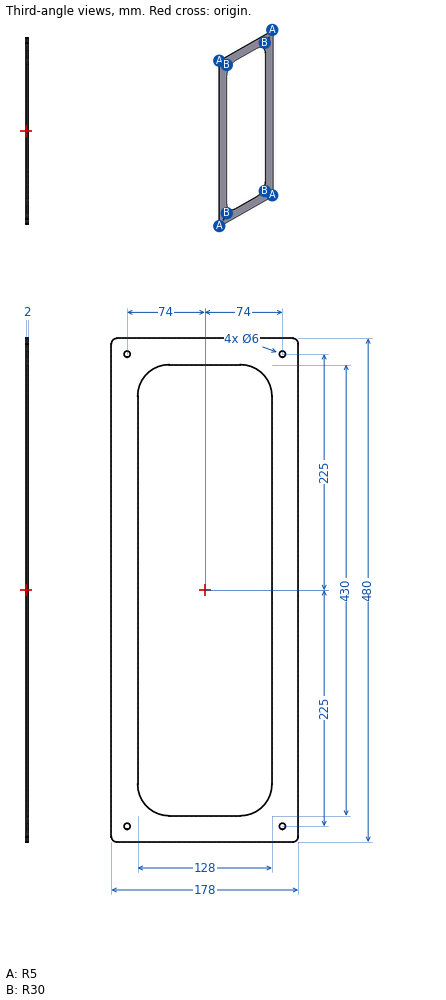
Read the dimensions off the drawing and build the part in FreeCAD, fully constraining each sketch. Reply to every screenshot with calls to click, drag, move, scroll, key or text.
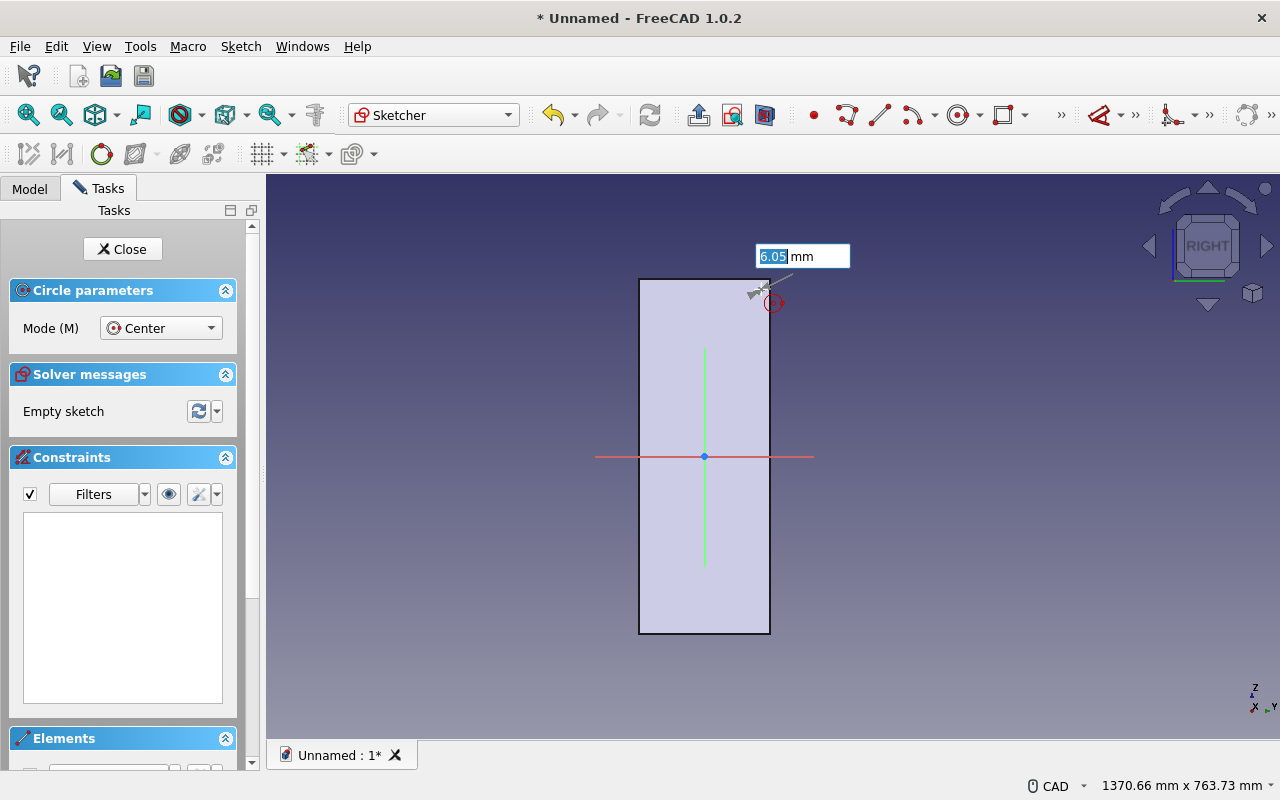
text(6)
key(Return)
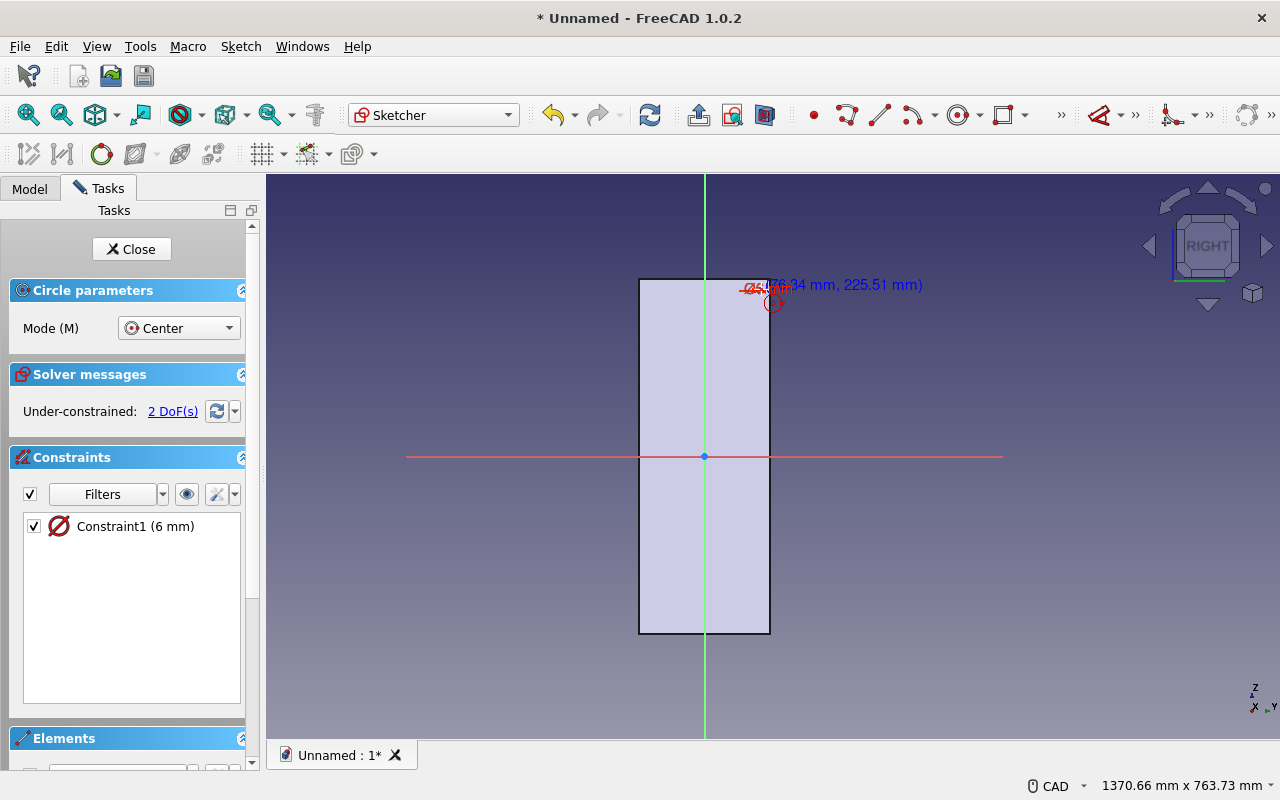
scroll(759, 623, up, 12)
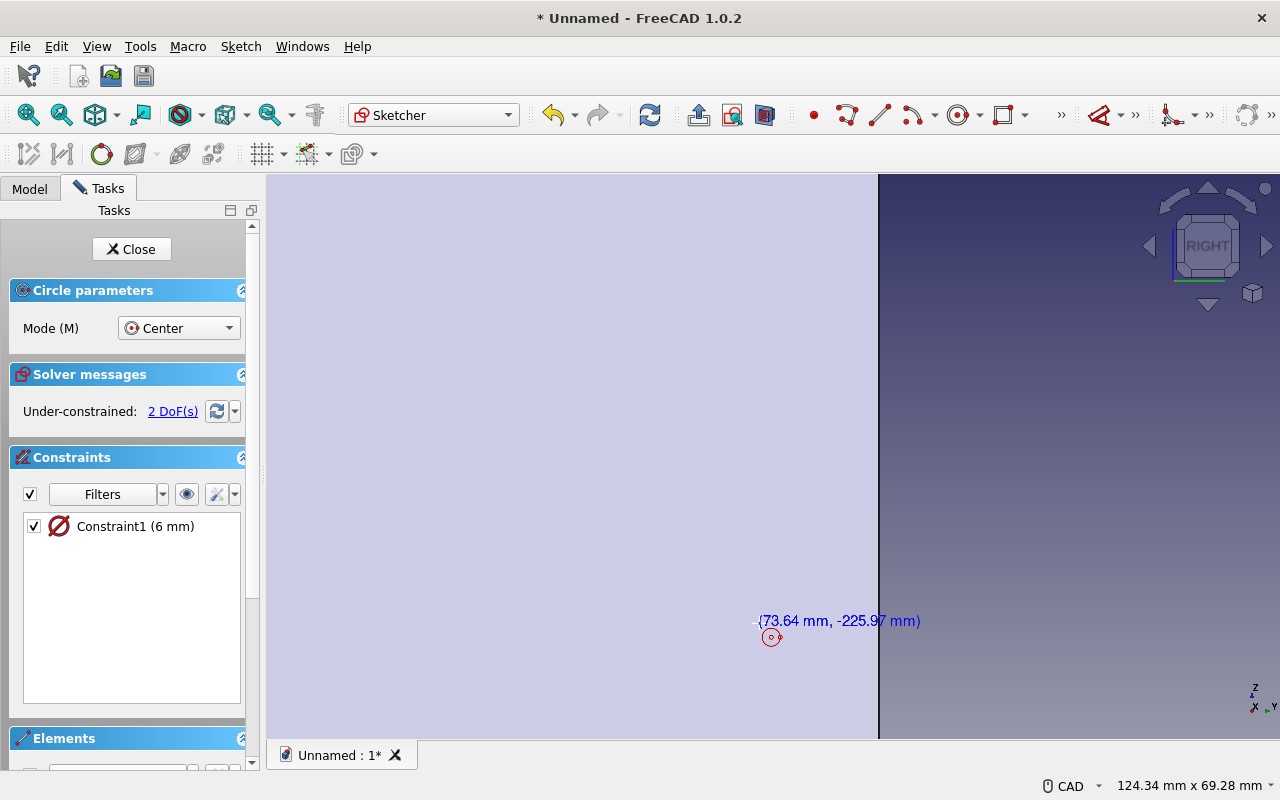
scroll(759, 623, down, 12)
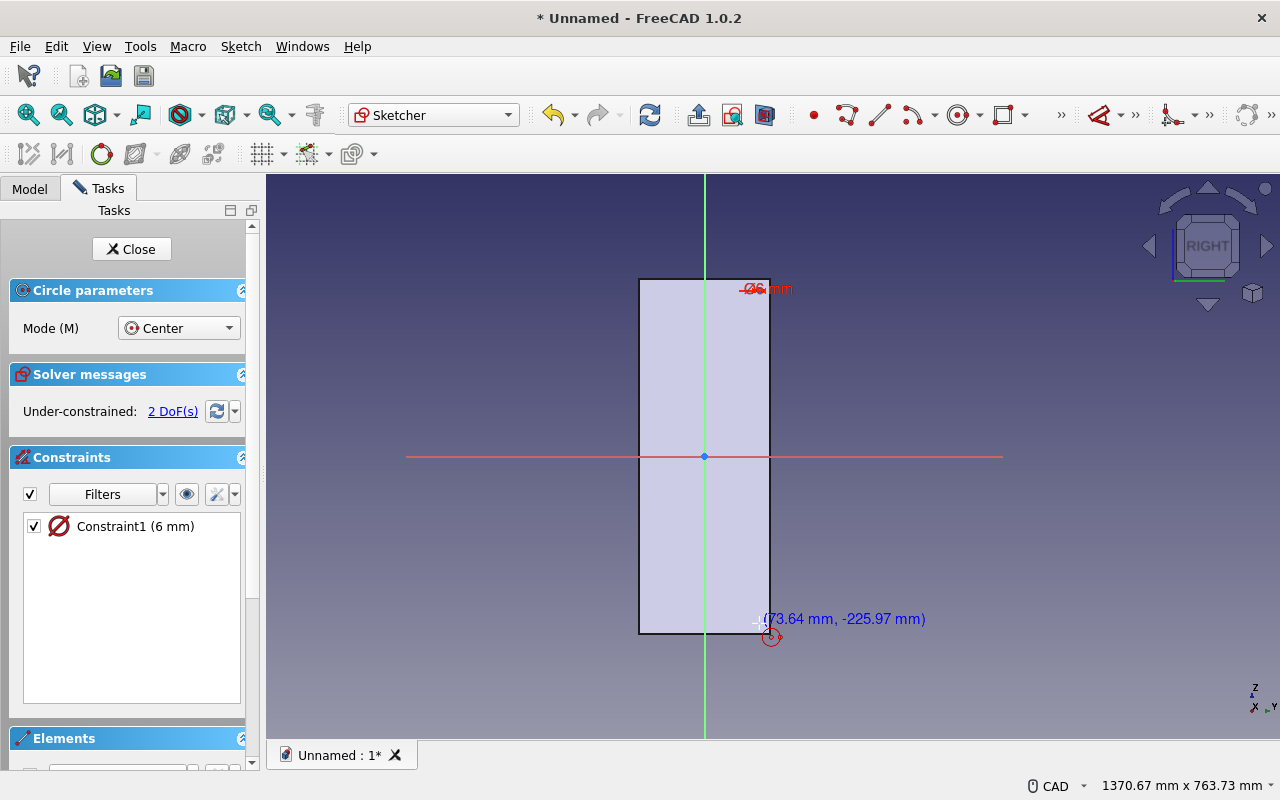
click(759, 623)
move(761, 622)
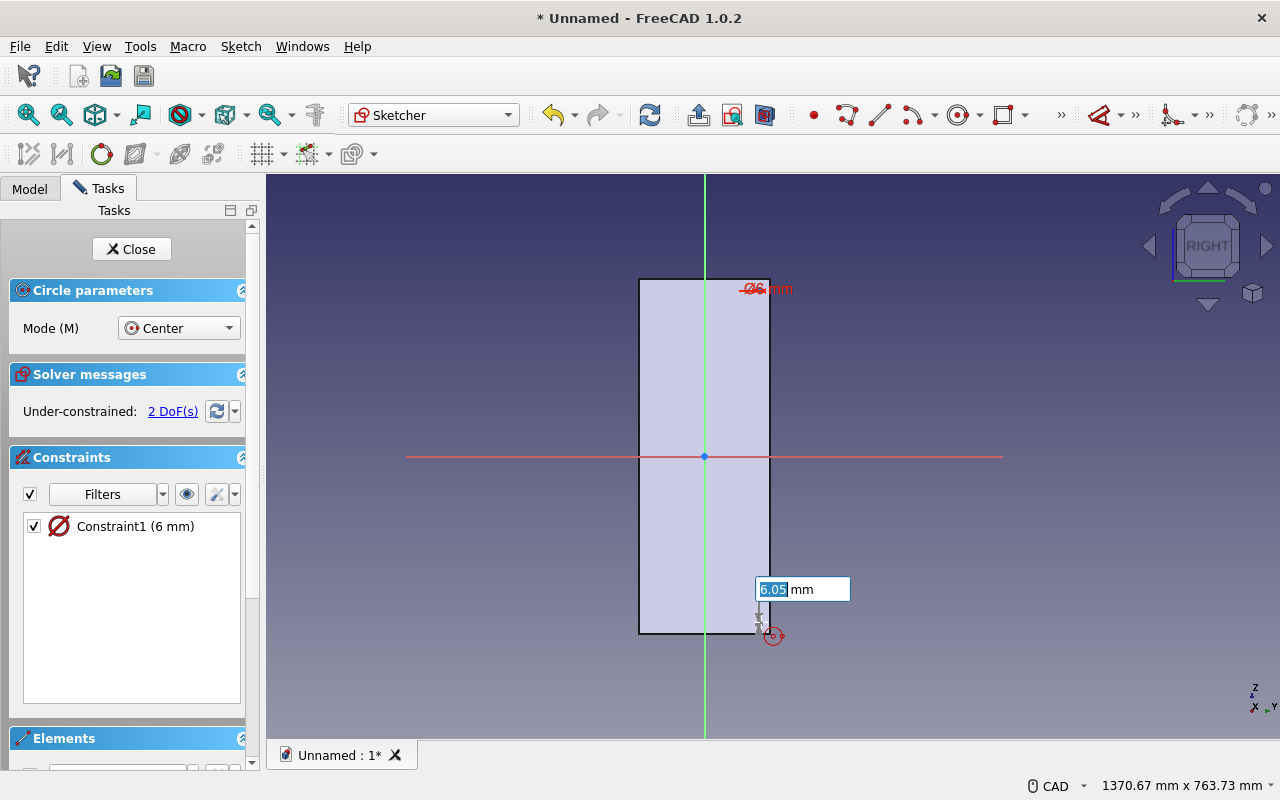
text(6)
key(Return)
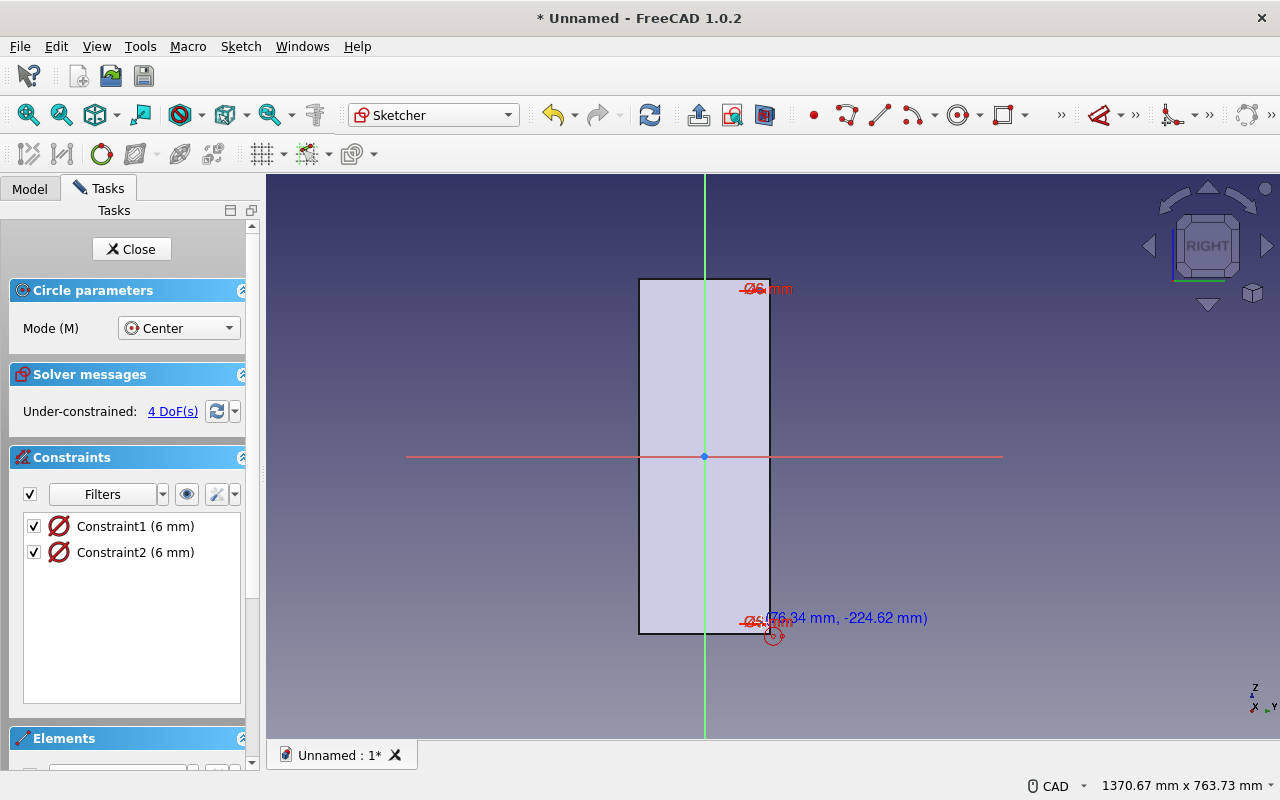
scroll(650, 290, up, 12)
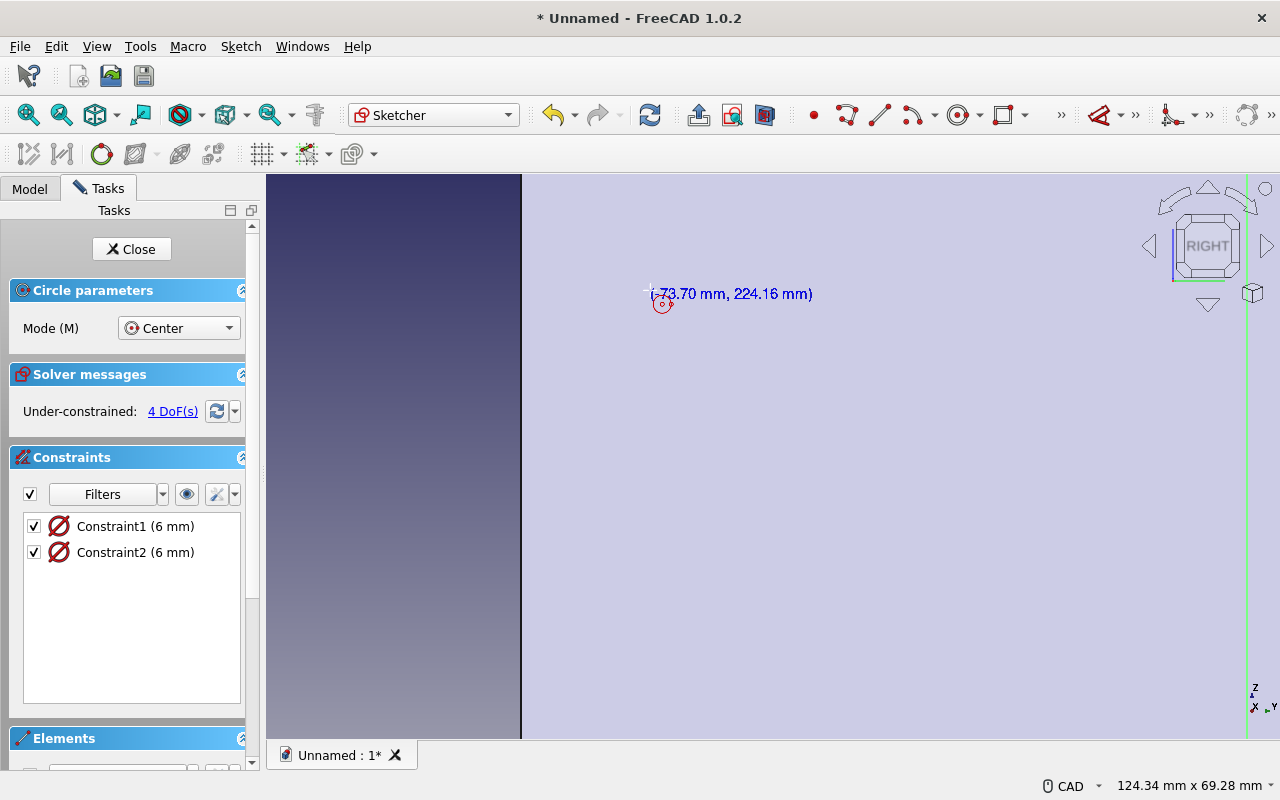
scroll(650, 290, down, 12)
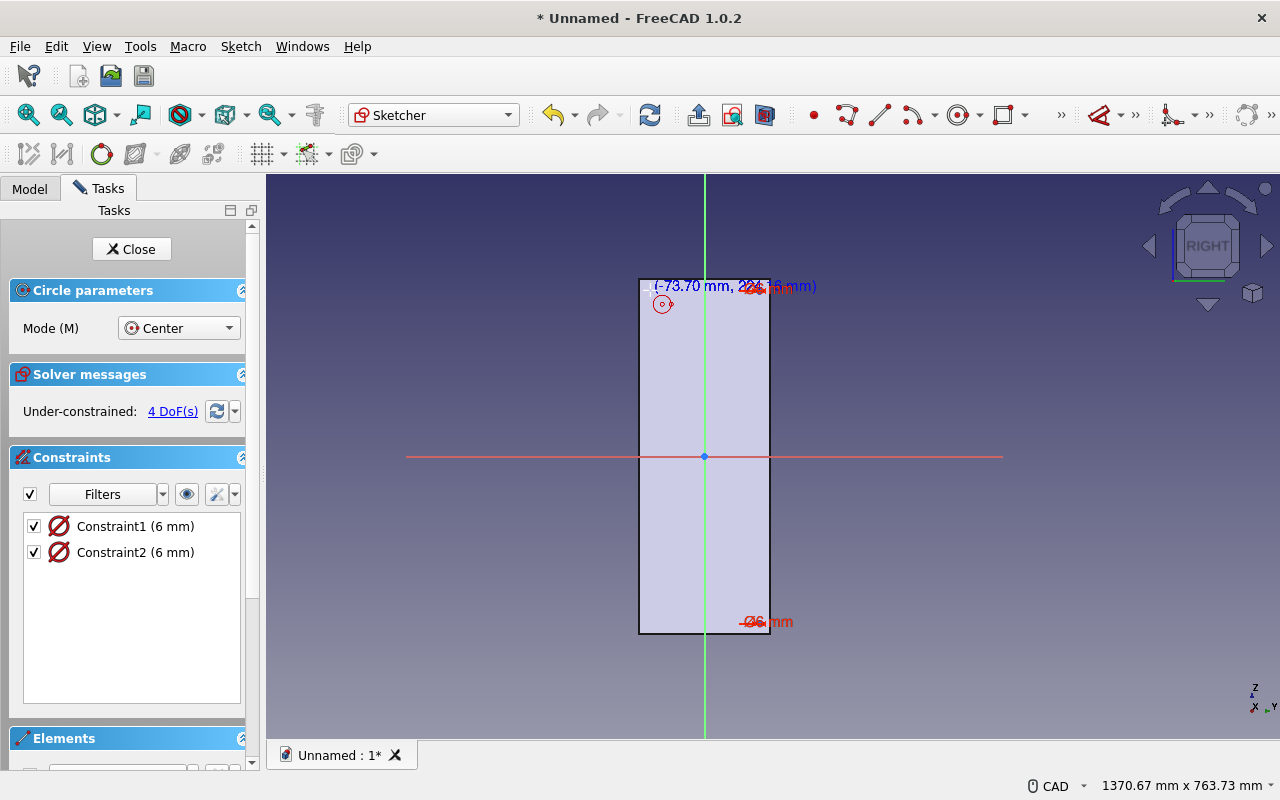
click(650, 290)
move(651, 289)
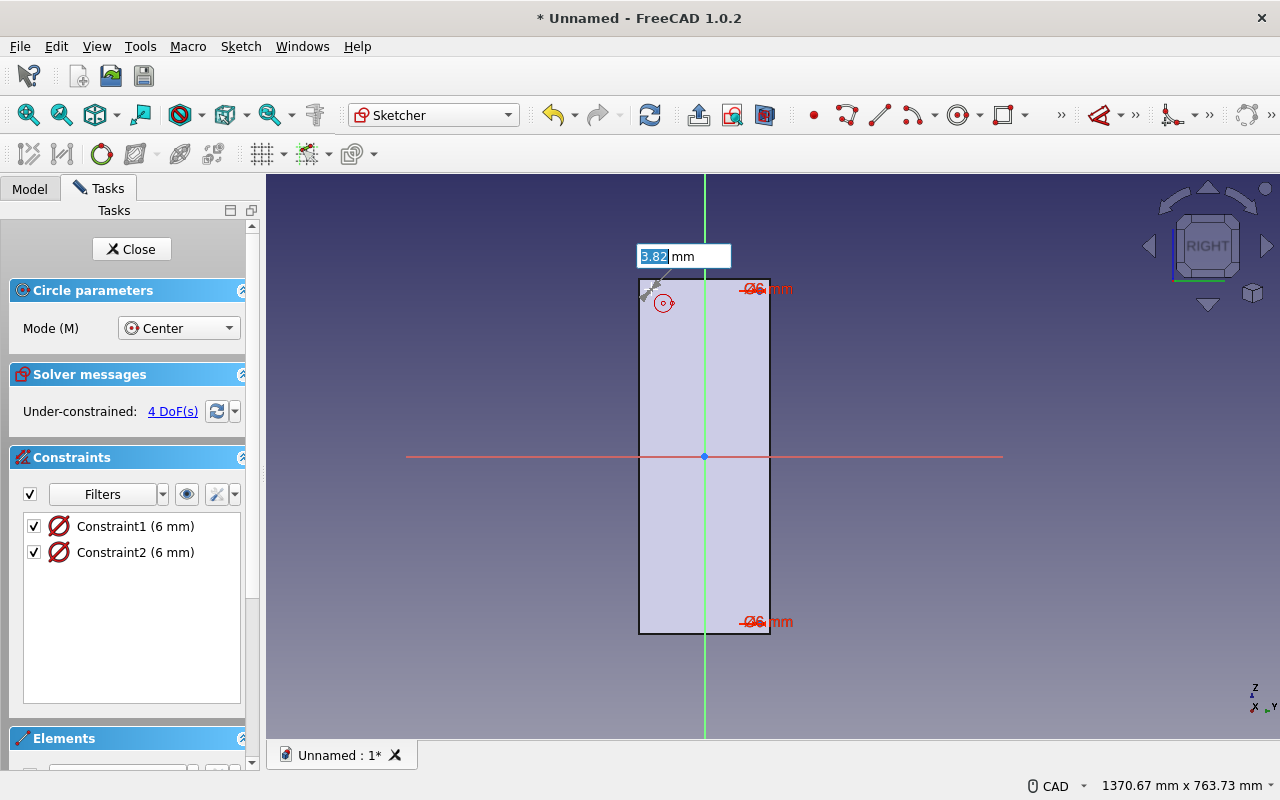
text(6)
key(Return)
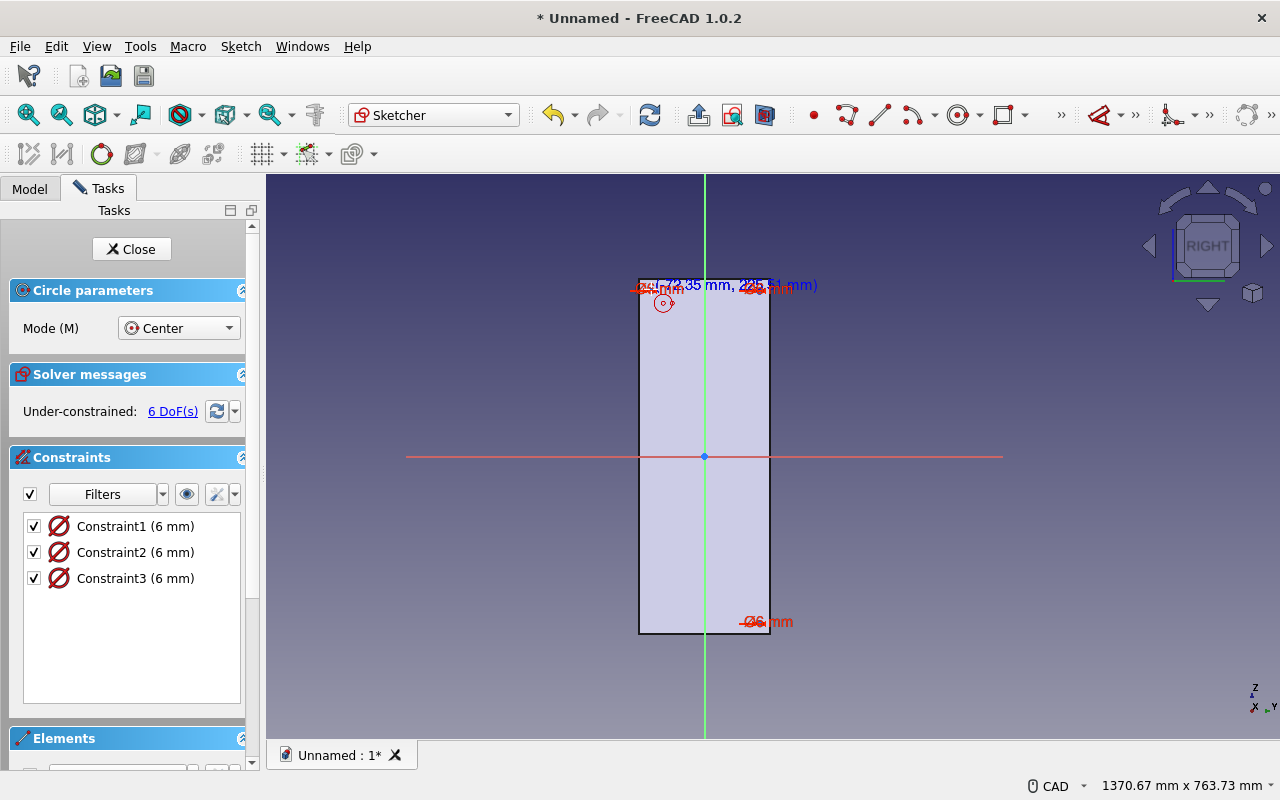
scroll(650, 623, up, 12)